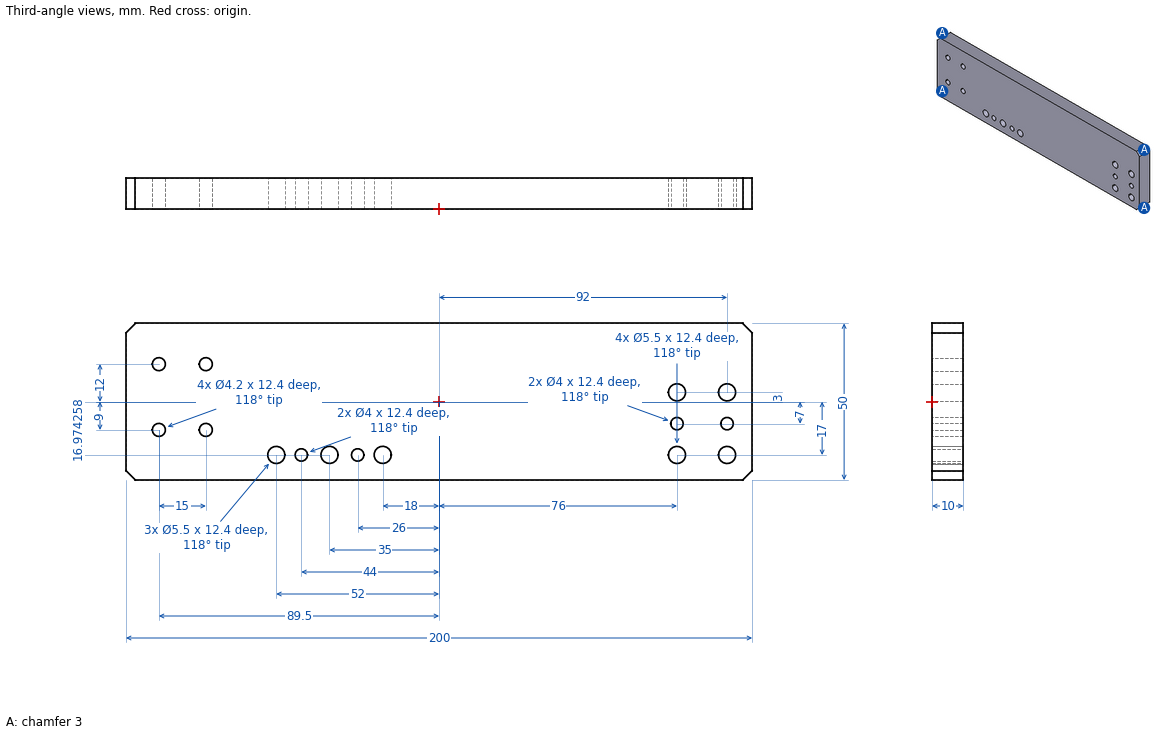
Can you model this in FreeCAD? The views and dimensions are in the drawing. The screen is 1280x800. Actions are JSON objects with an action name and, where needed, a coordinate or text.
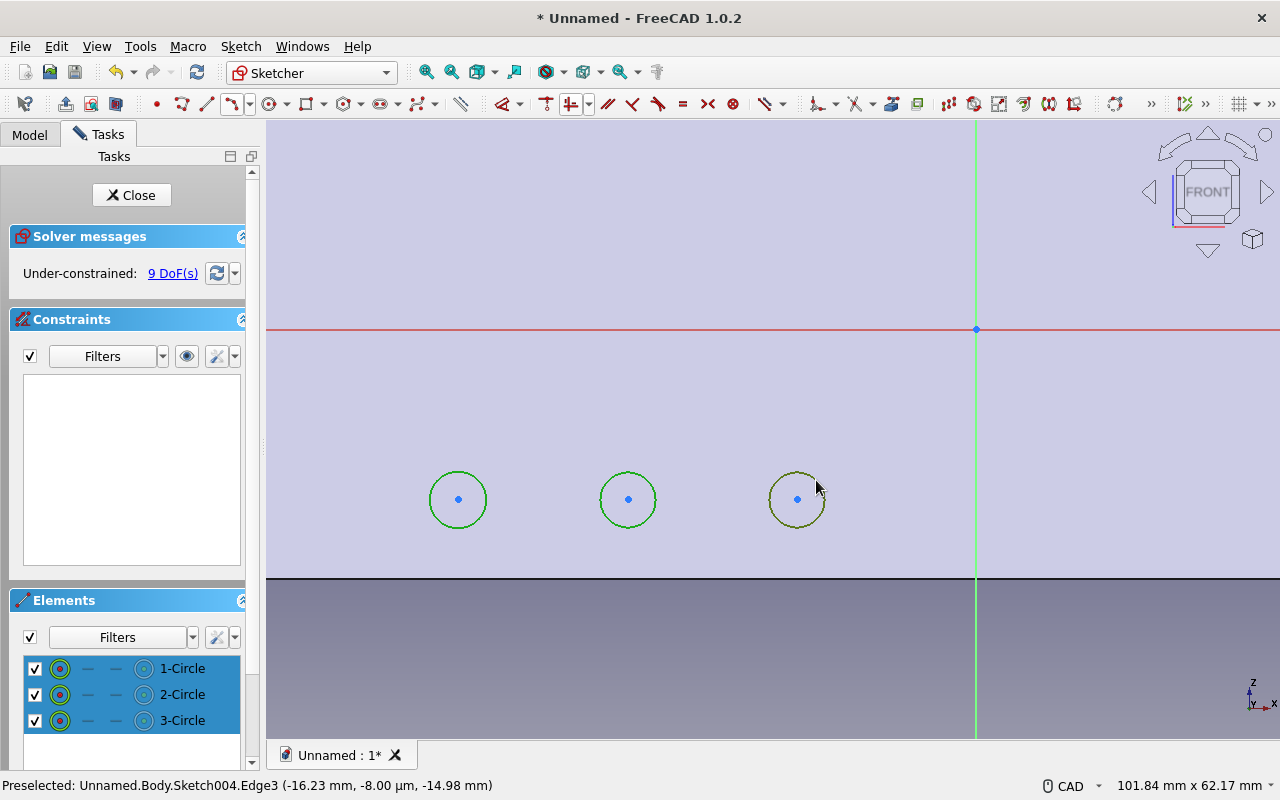
{"action": "key", "text": "e"}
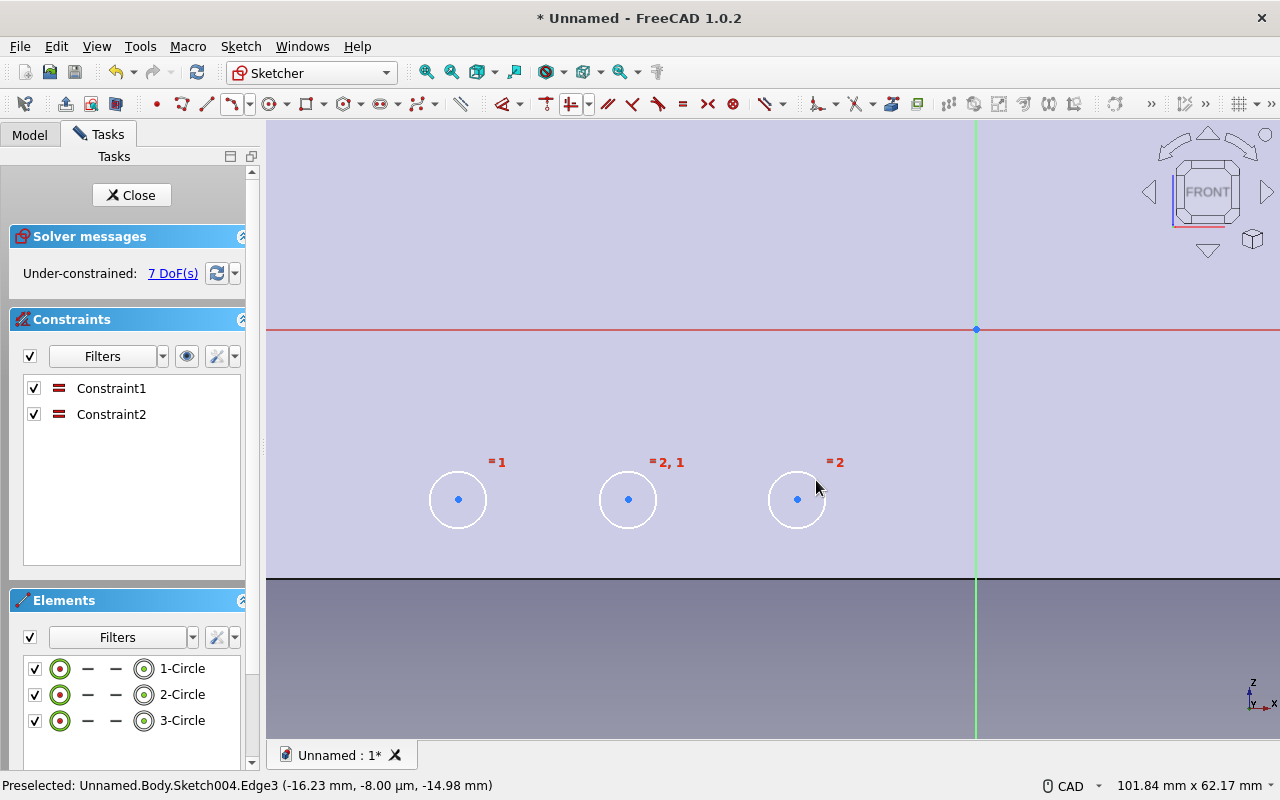
{"action": "left_click", "coordinate": [628, 500]}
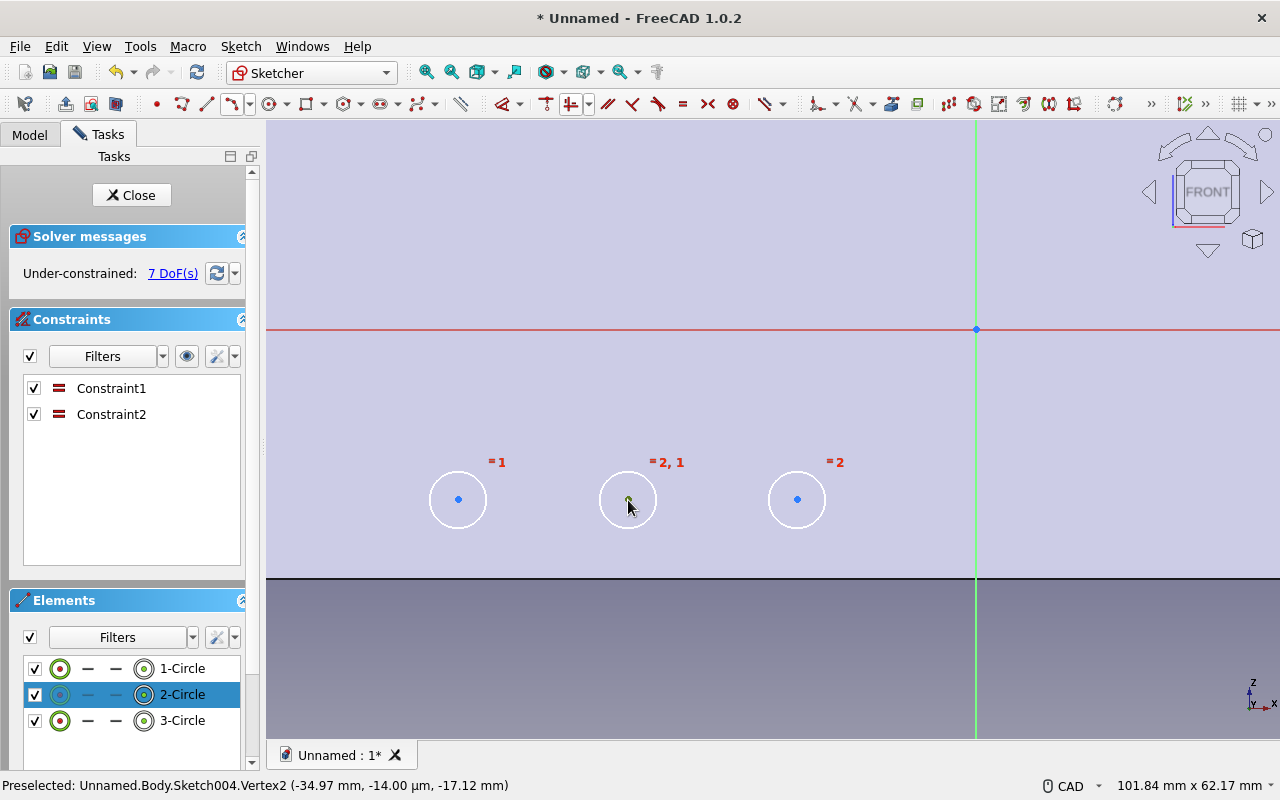
{"action": "left_click", "coordinate": [797, 500]}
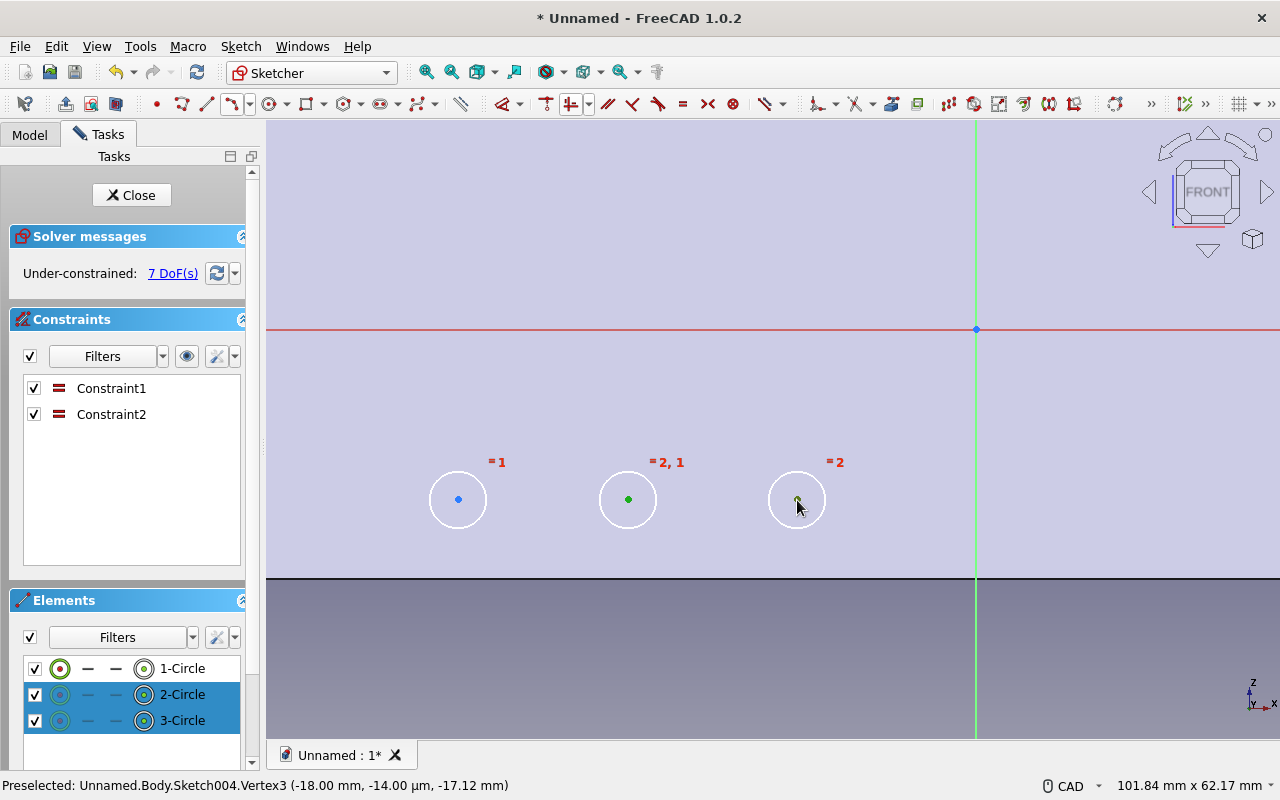
{"action": "key", "text": "h"}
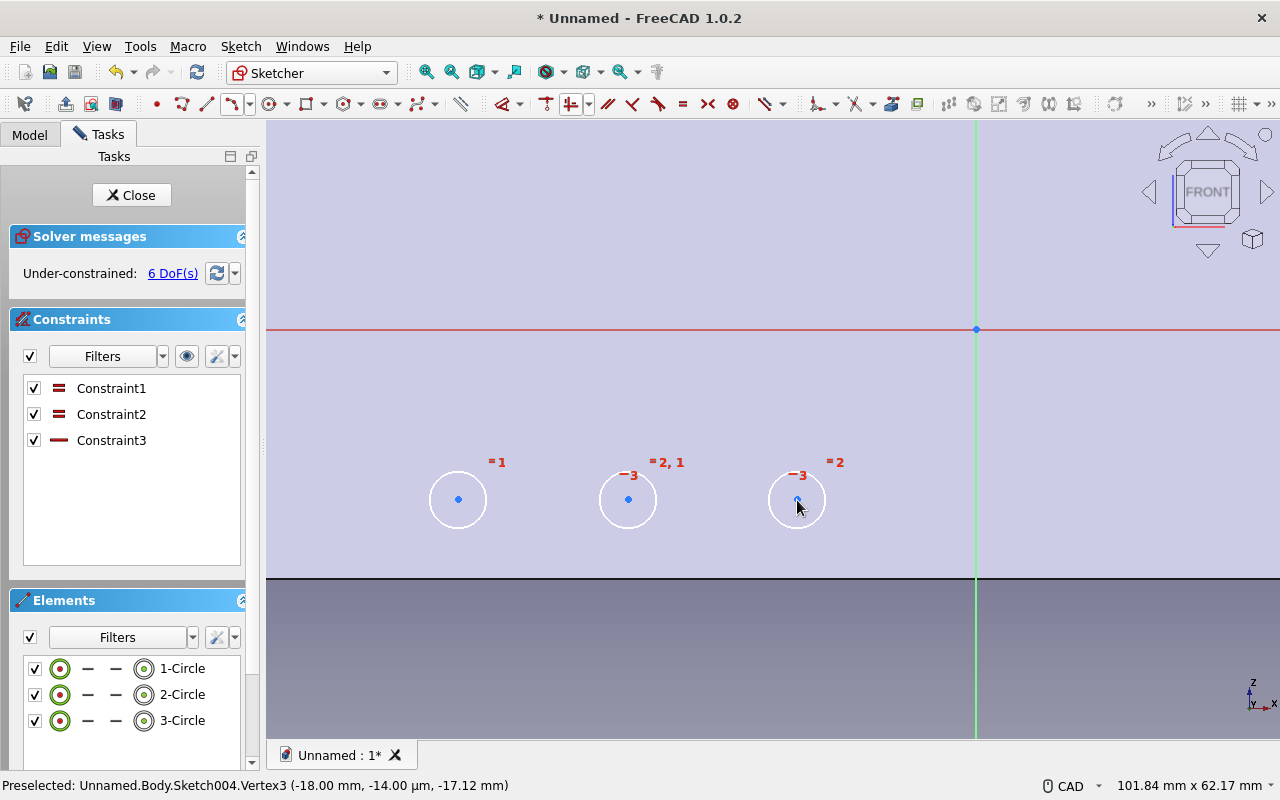
{"action": "left_click", "coordinate": [502, 104]}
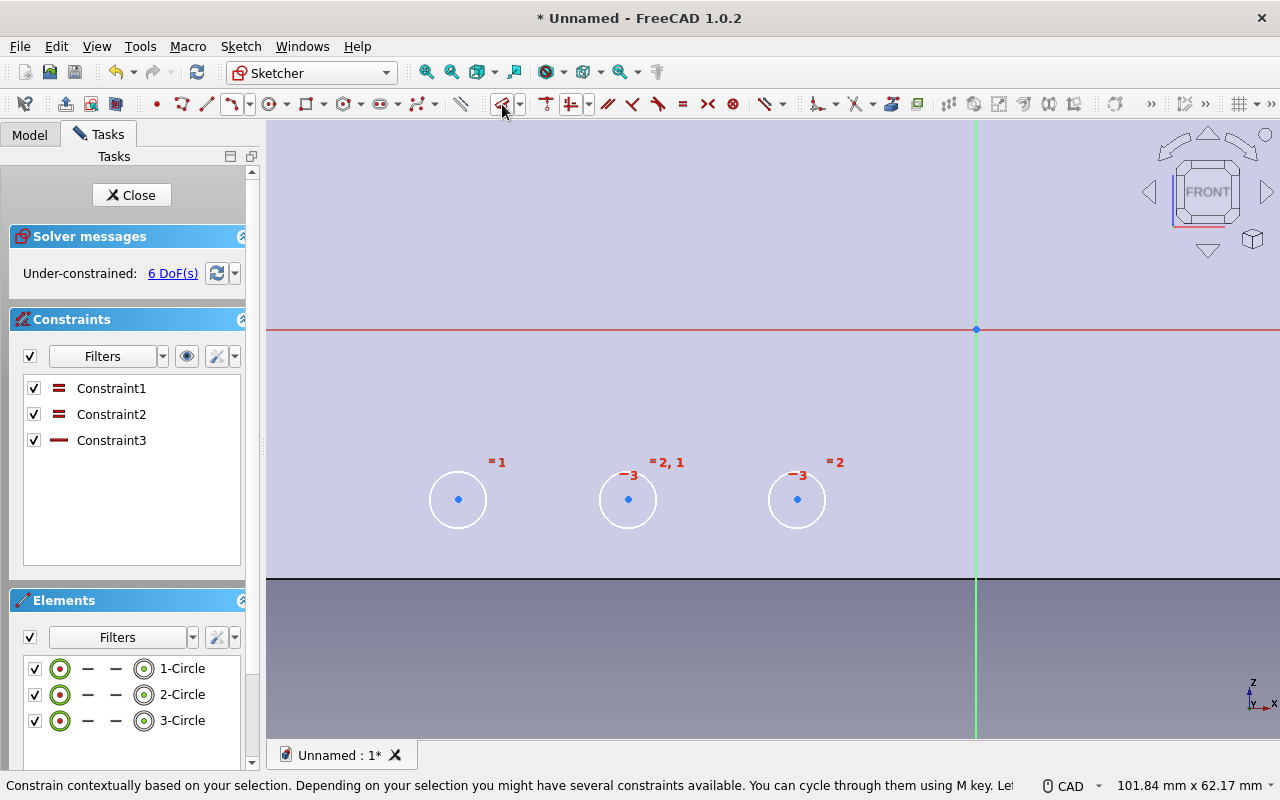
{"action": "left_click", "coordinate": [478, 480]}
{"action": "left_click", "coordinate": [501, 457]}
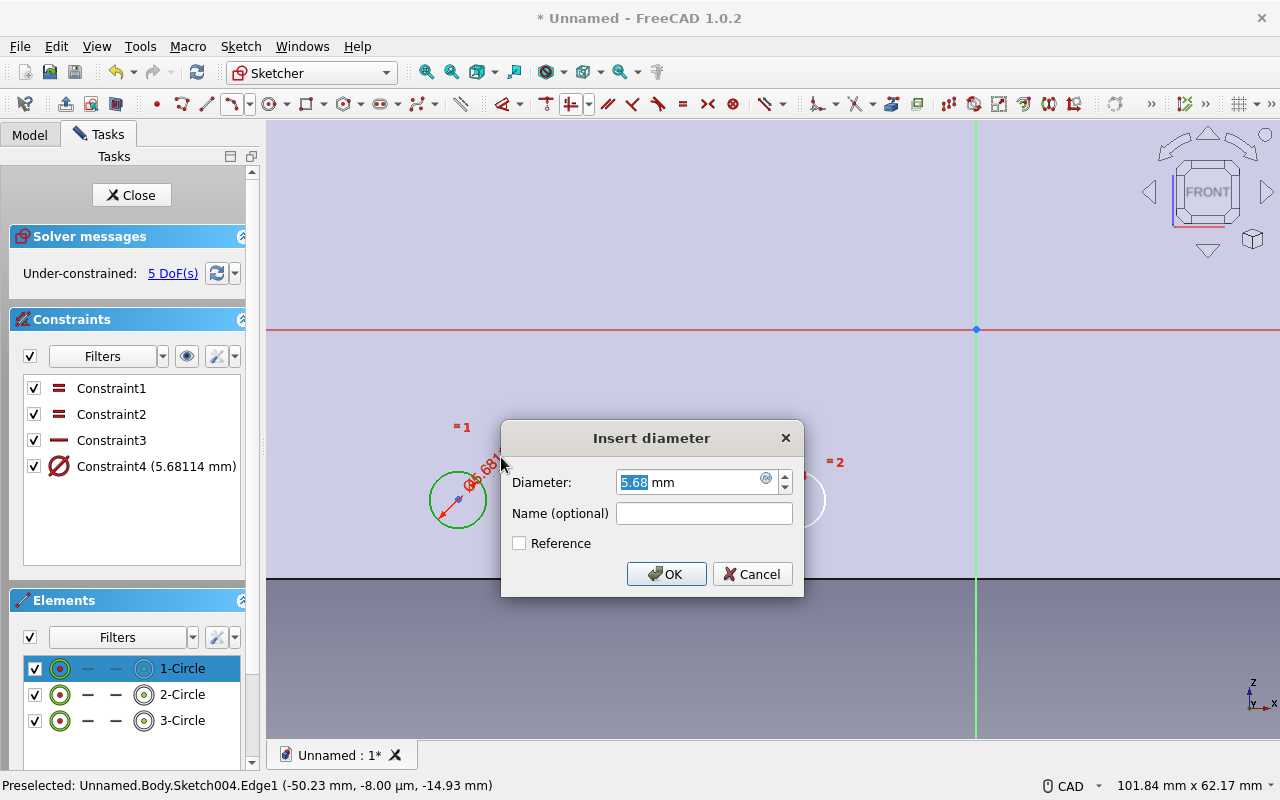
{"action": "type", "text": "5.5"}
{"action": "key", "text": "Return"}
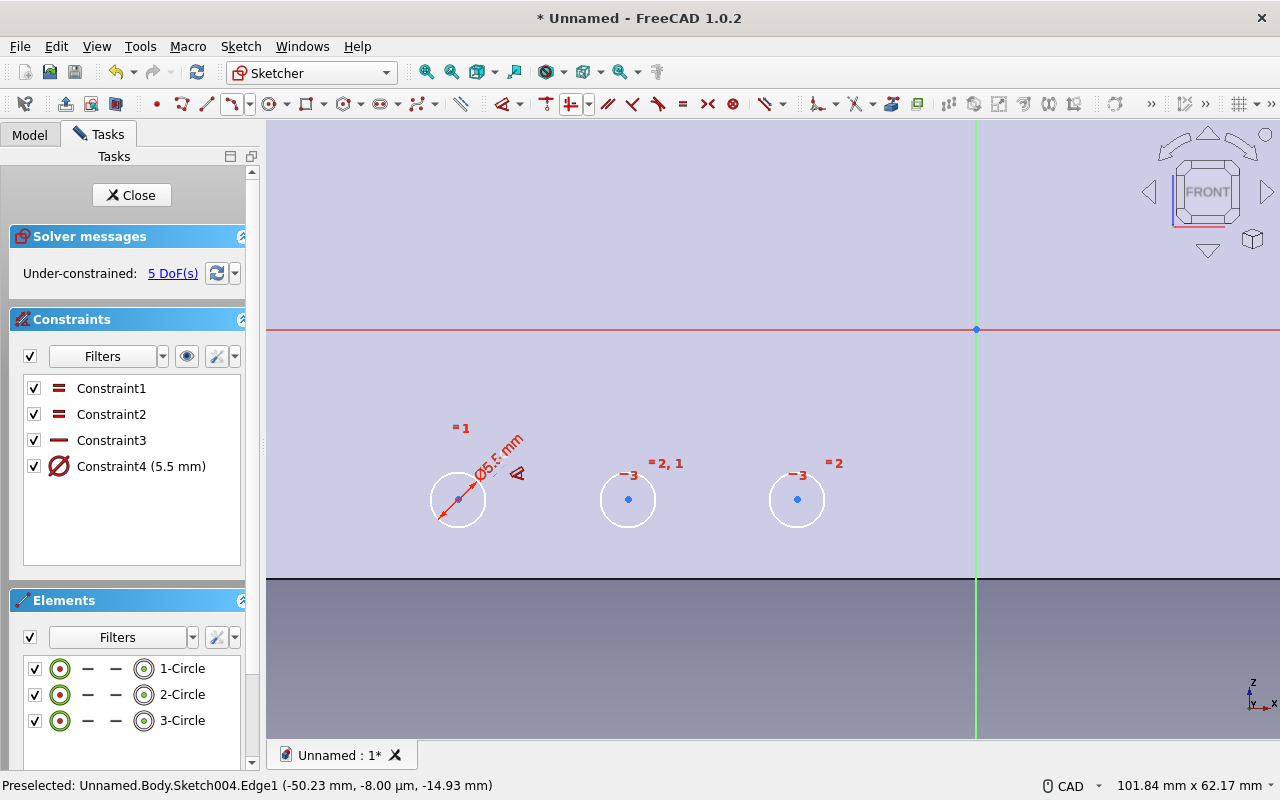
{"action": "left_click", "coordinate": [458, 500]}
{"action": "left_click", "coordinate": [717, 296]}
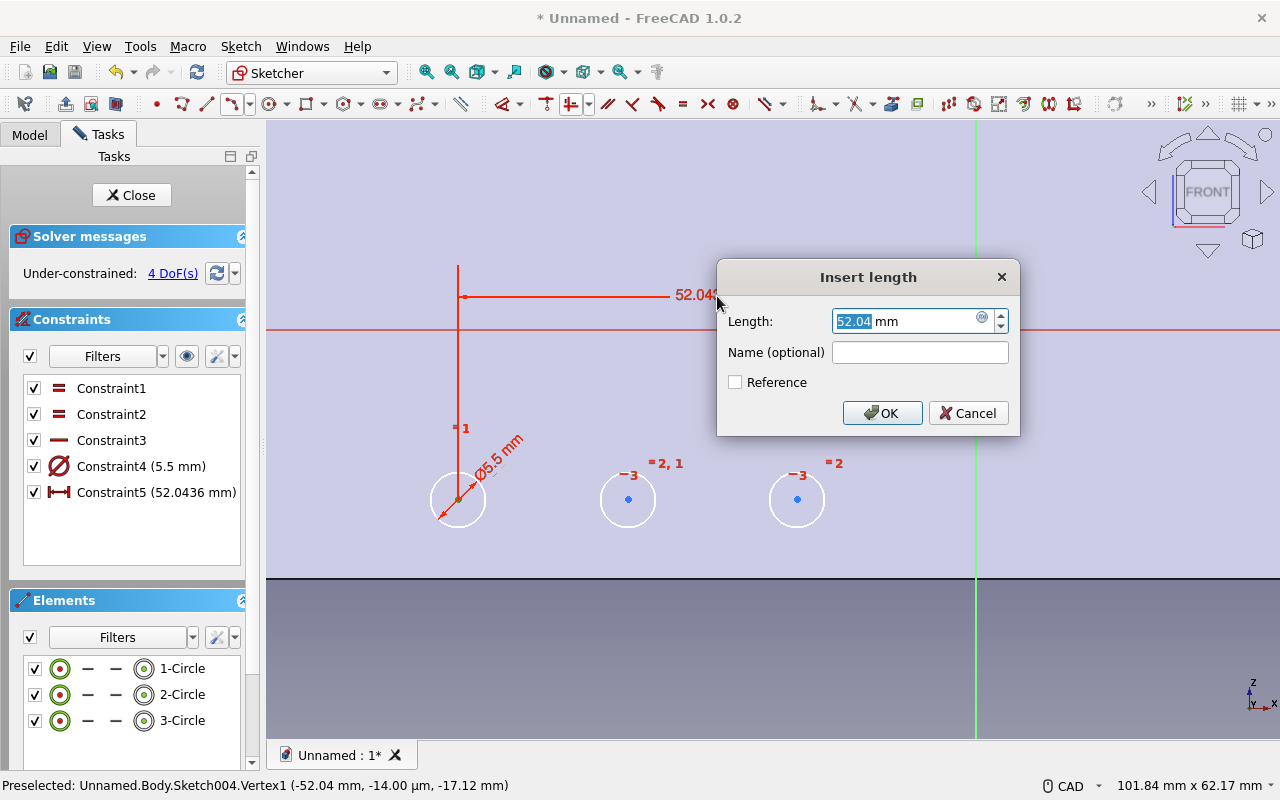
{"action": "type", "text": "52"}
{"action": "key", "text": "Return"}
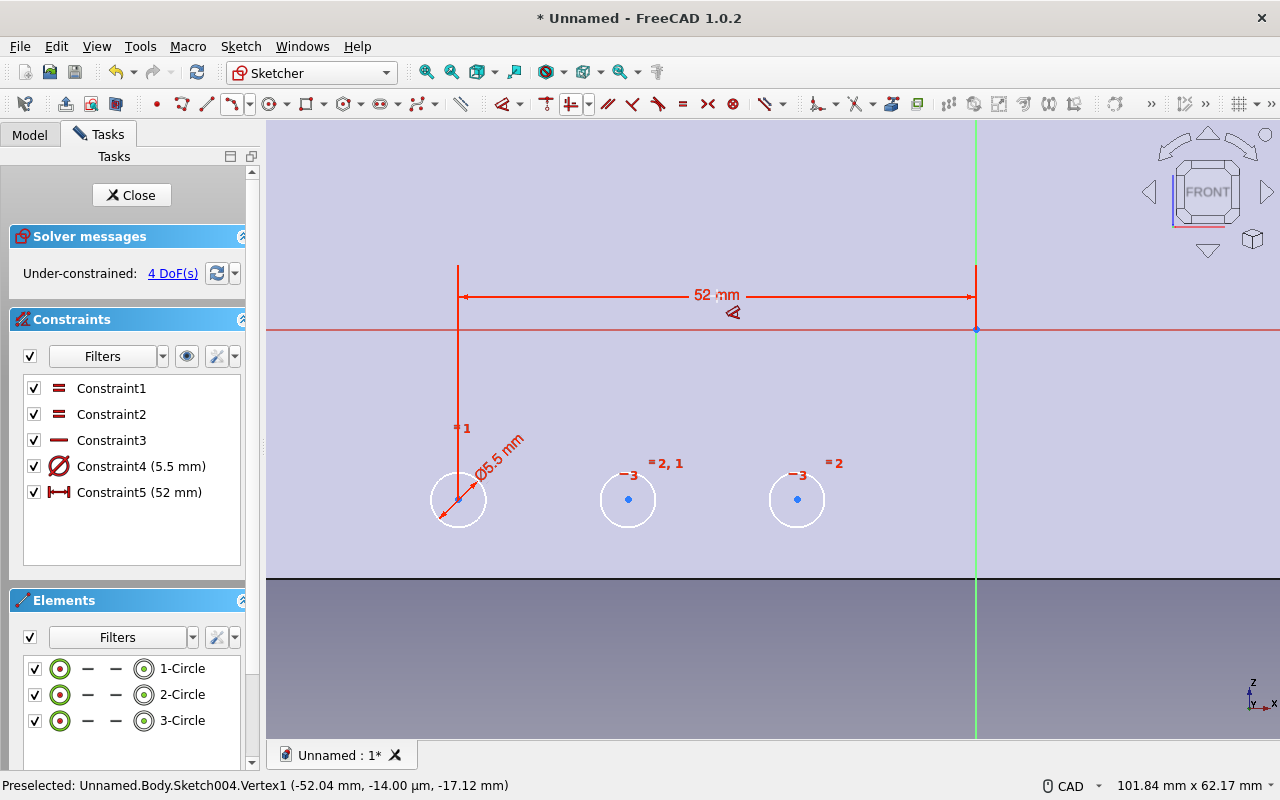
{"action": "left_click", "coordinate": [458, 500]}
{"action": "left_click", "coordinate": [1010, 415]}